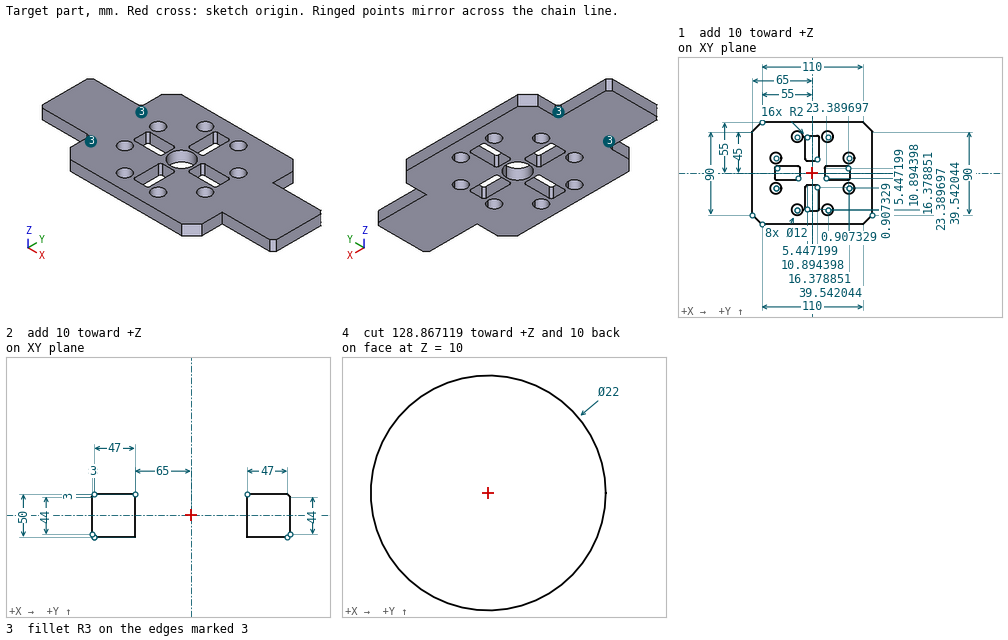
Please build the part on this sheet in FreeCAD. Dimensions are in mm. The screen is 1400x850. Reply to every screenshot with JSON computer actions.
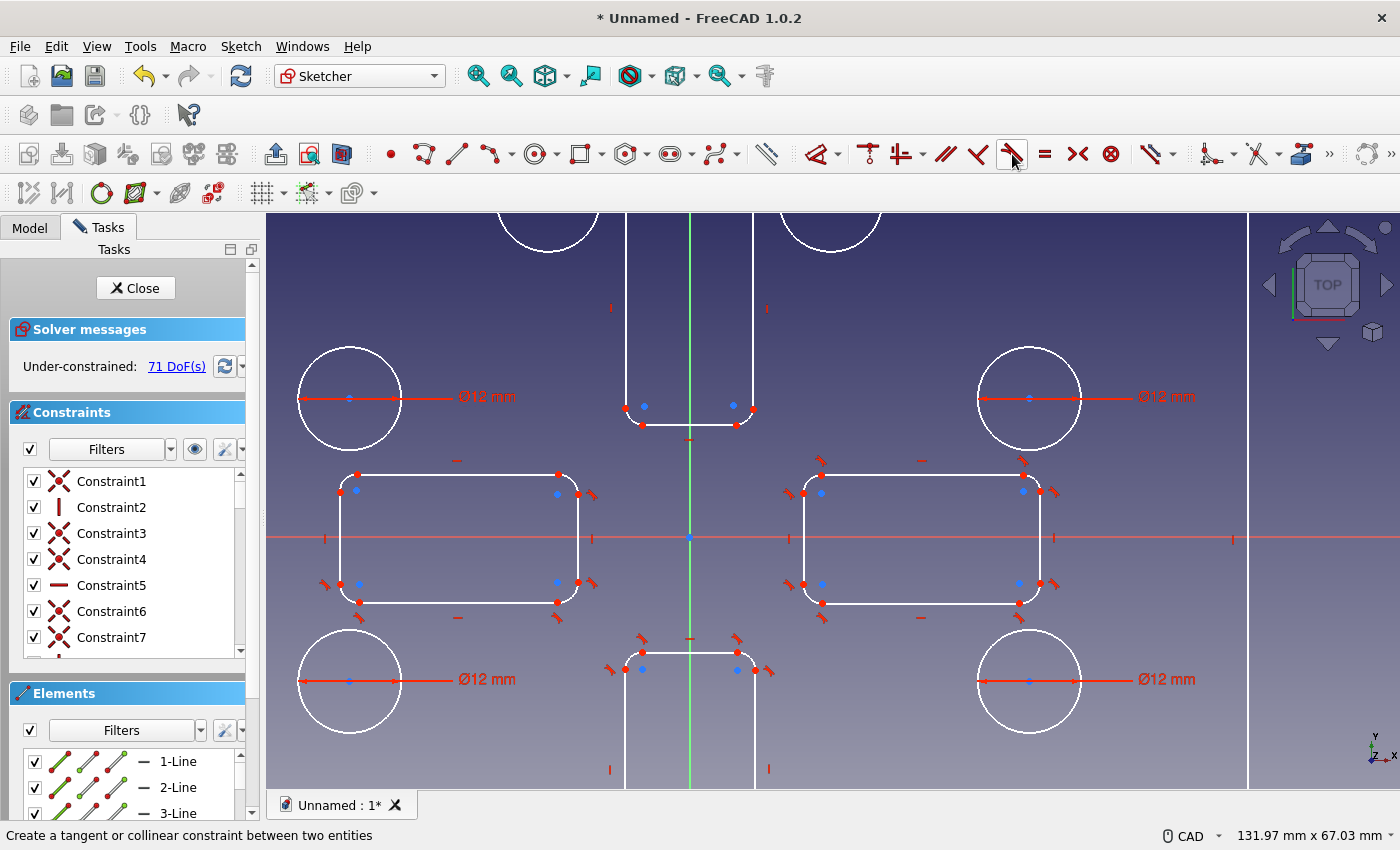
{"action": "left_click", "coordinate": [340, 557]}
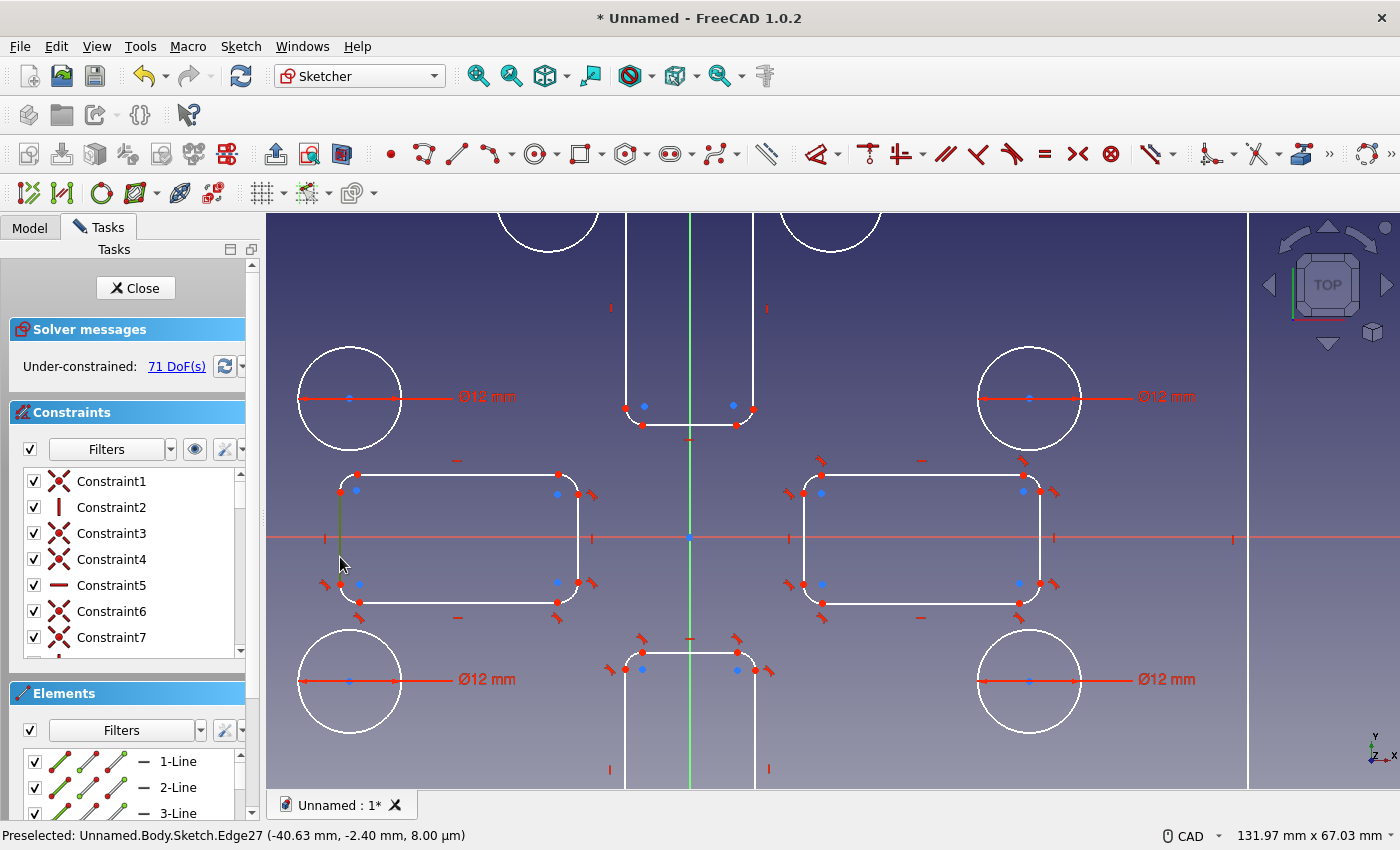
{"action": "left_click", "coordinate": [345, 480]}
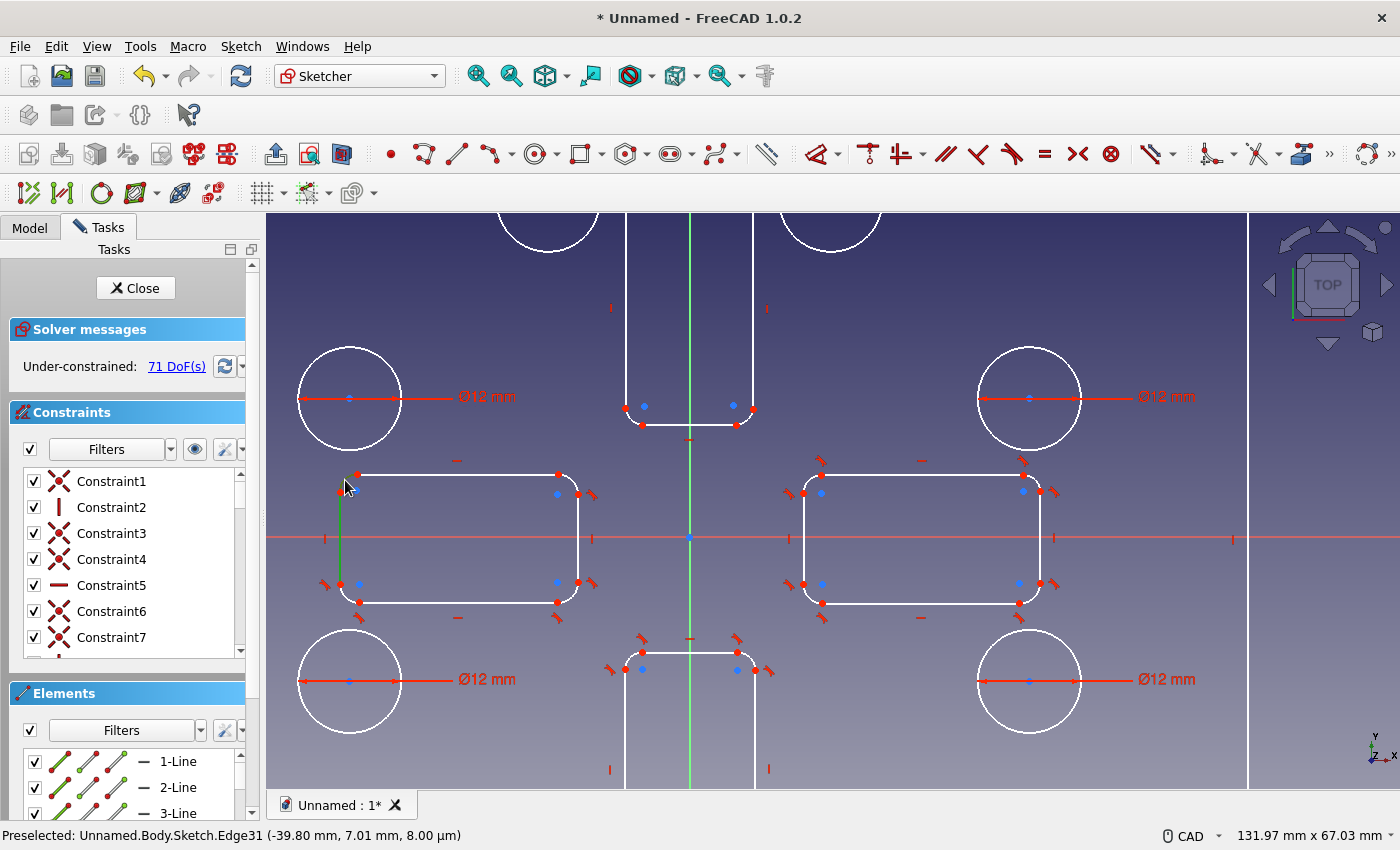
{"action": "left_click", "coordinate": [1012, 154]}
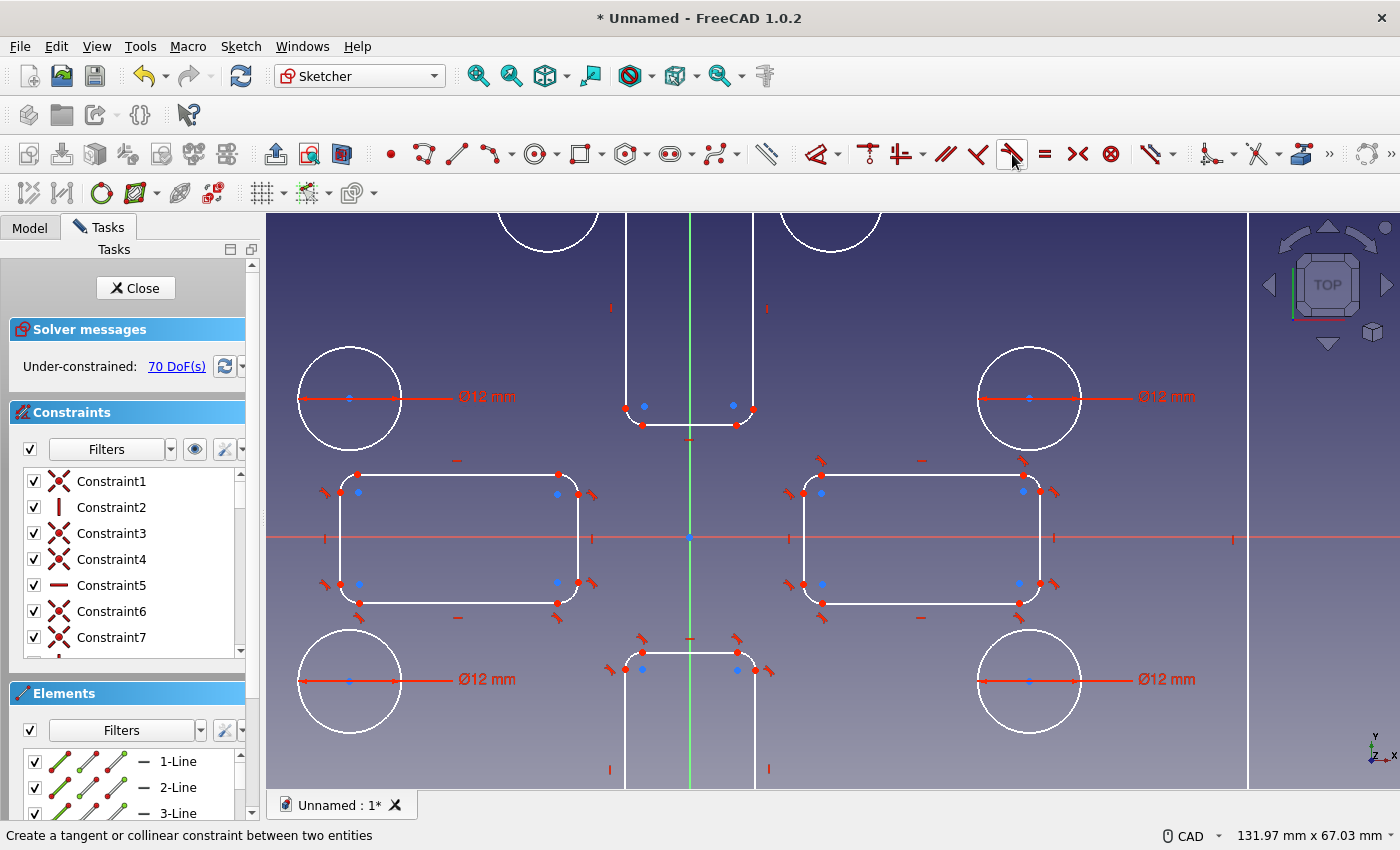
{"action": "left_click", "coordinate": [417, 475]}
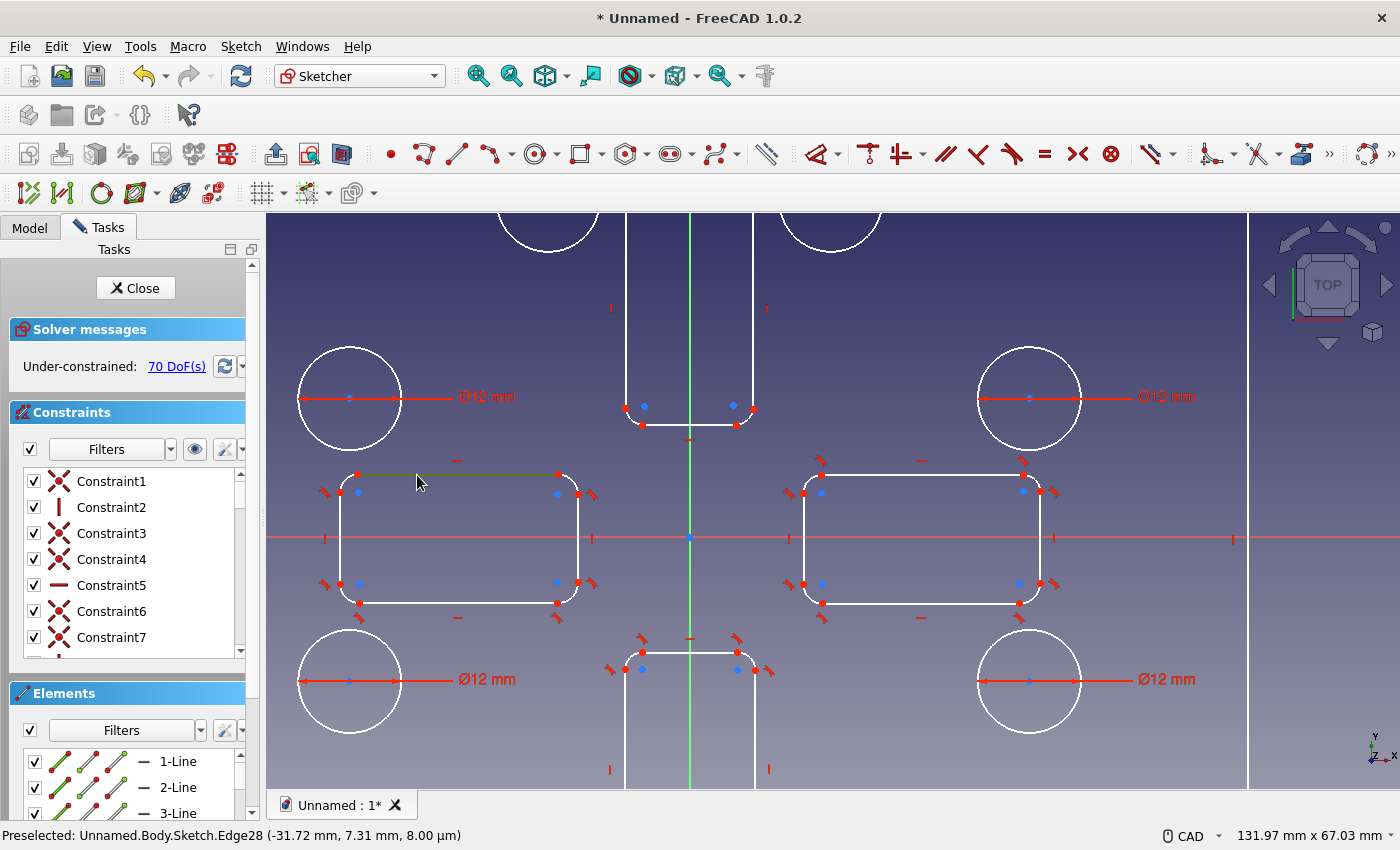
{"action": "left_click", "coordinate": [345, 480]}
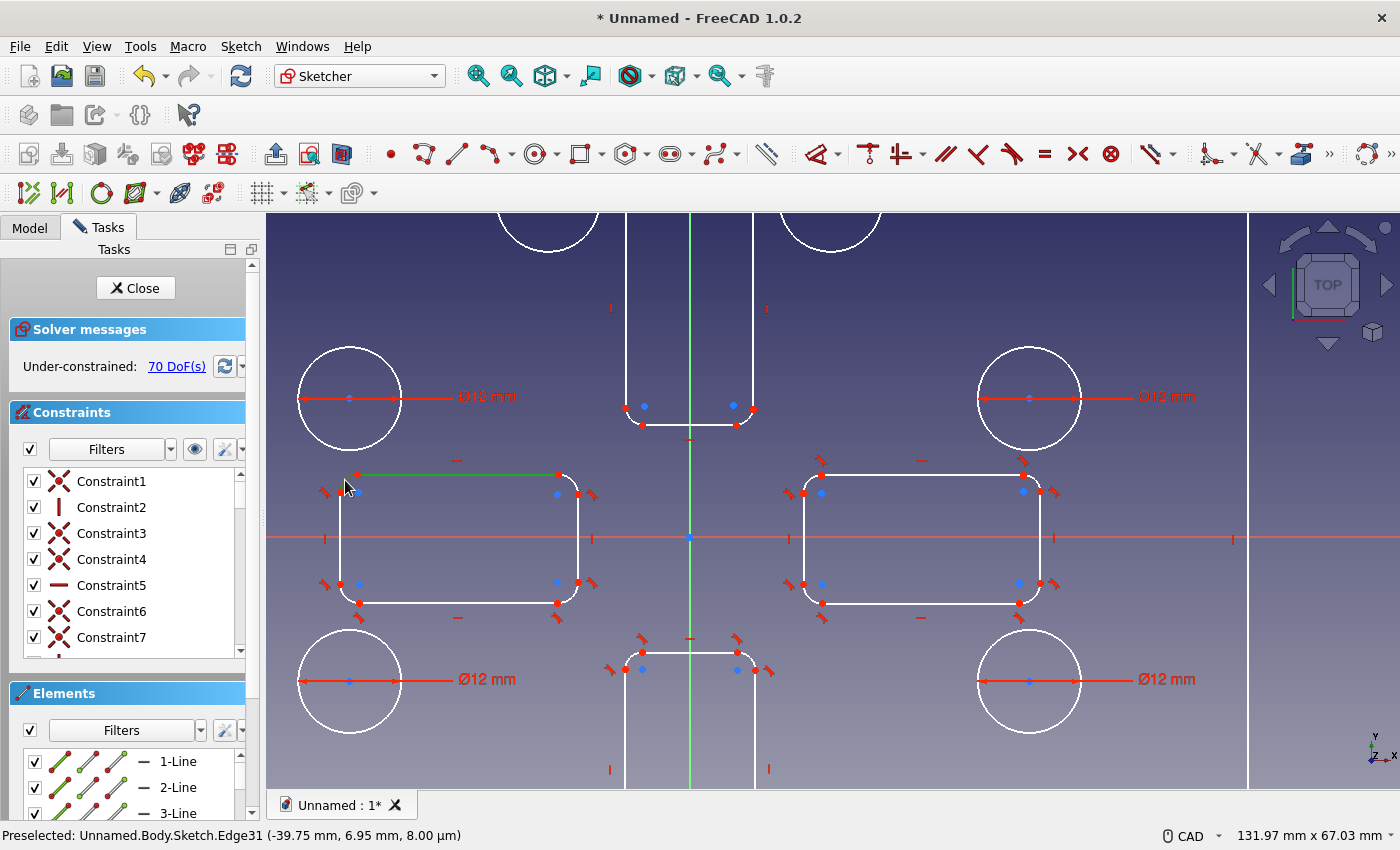
{"action": "left_click", "coordinate": [1012, 154]}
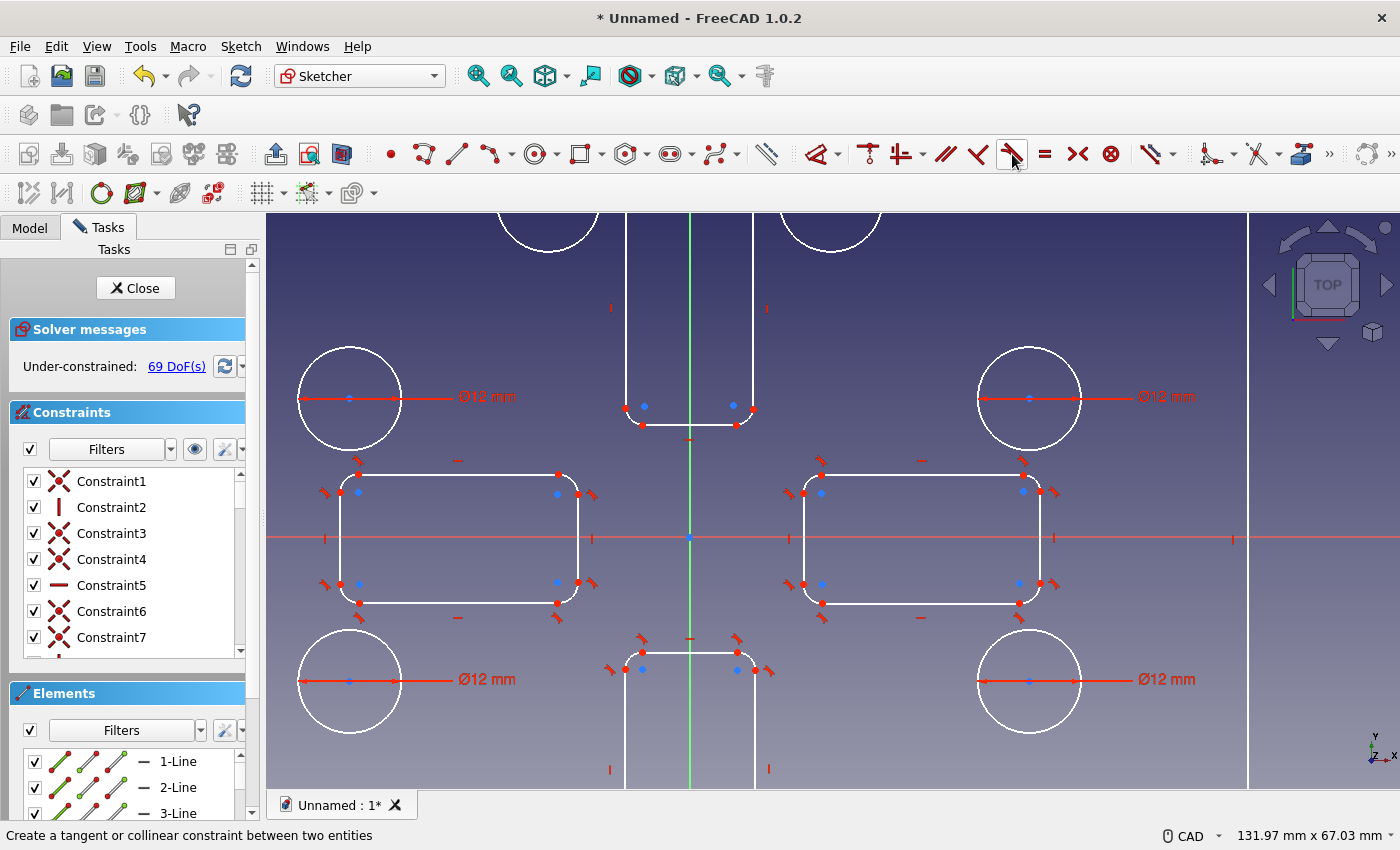
{"action": "left_click", "coordinate": [418, 475]}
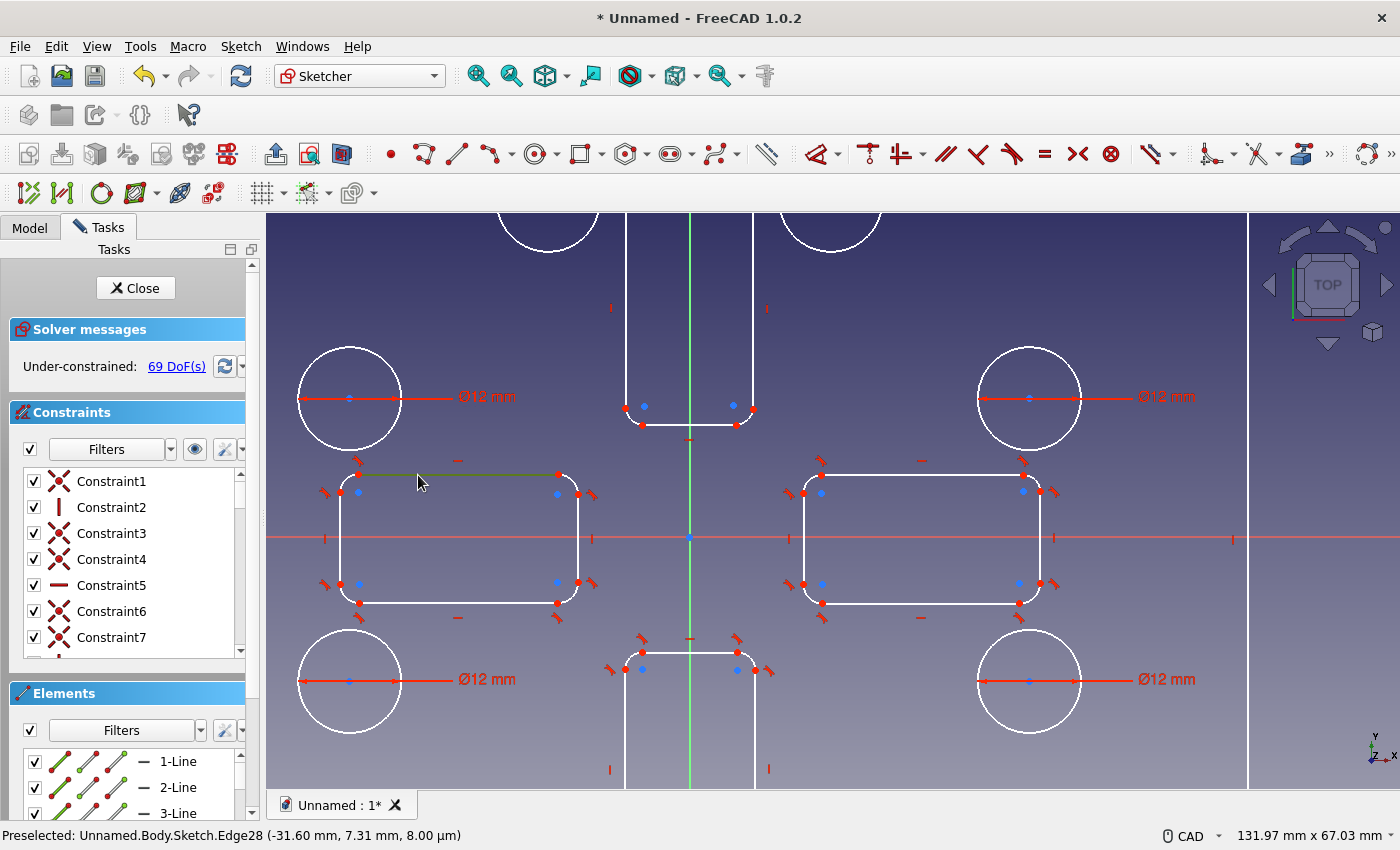
{"action": "scroll", "coordinate": [576, 486], "scroll_direction": "up", "scroll_amount": 3}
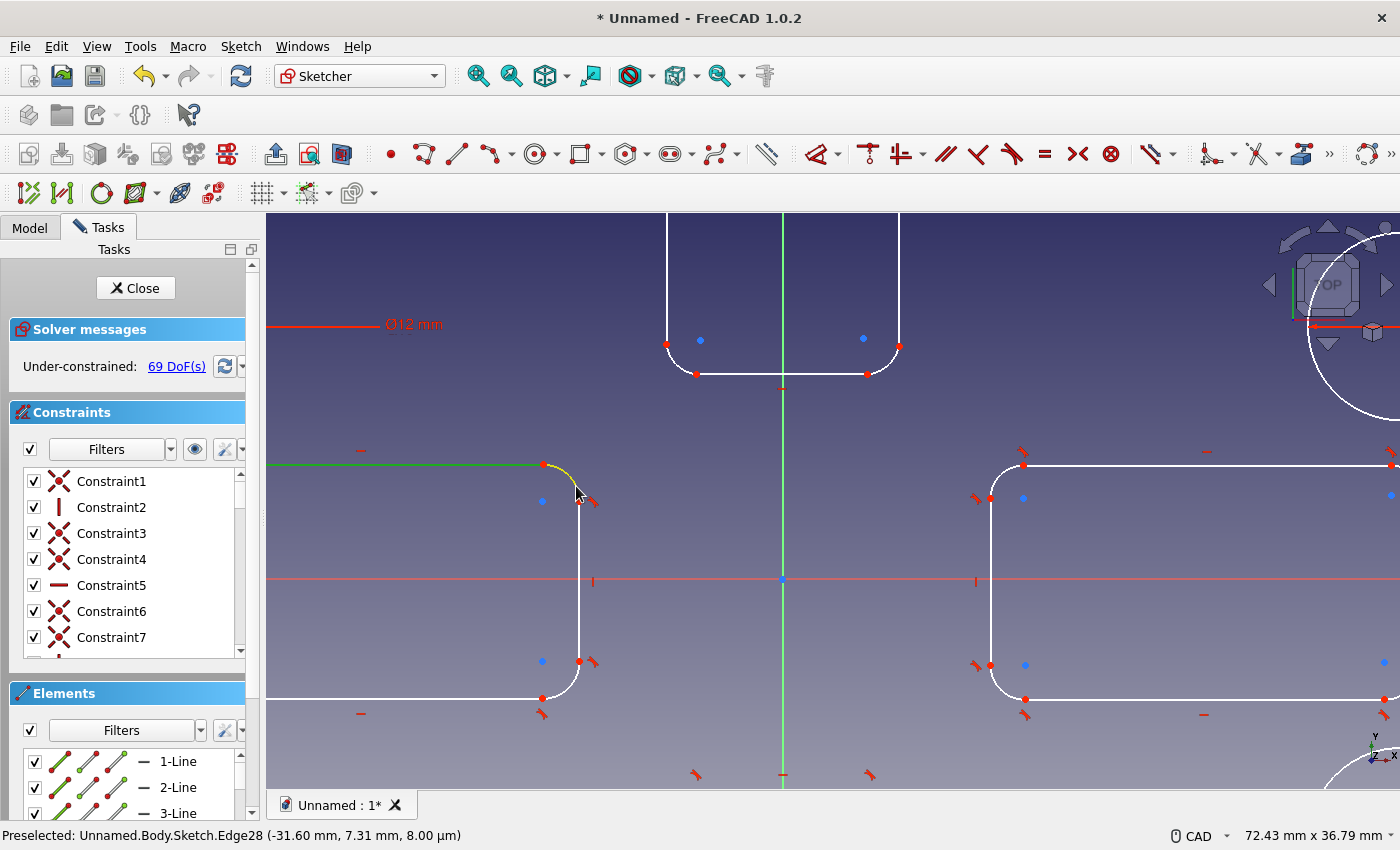
{"action": "left_click", "coordinate": [576, 485]}